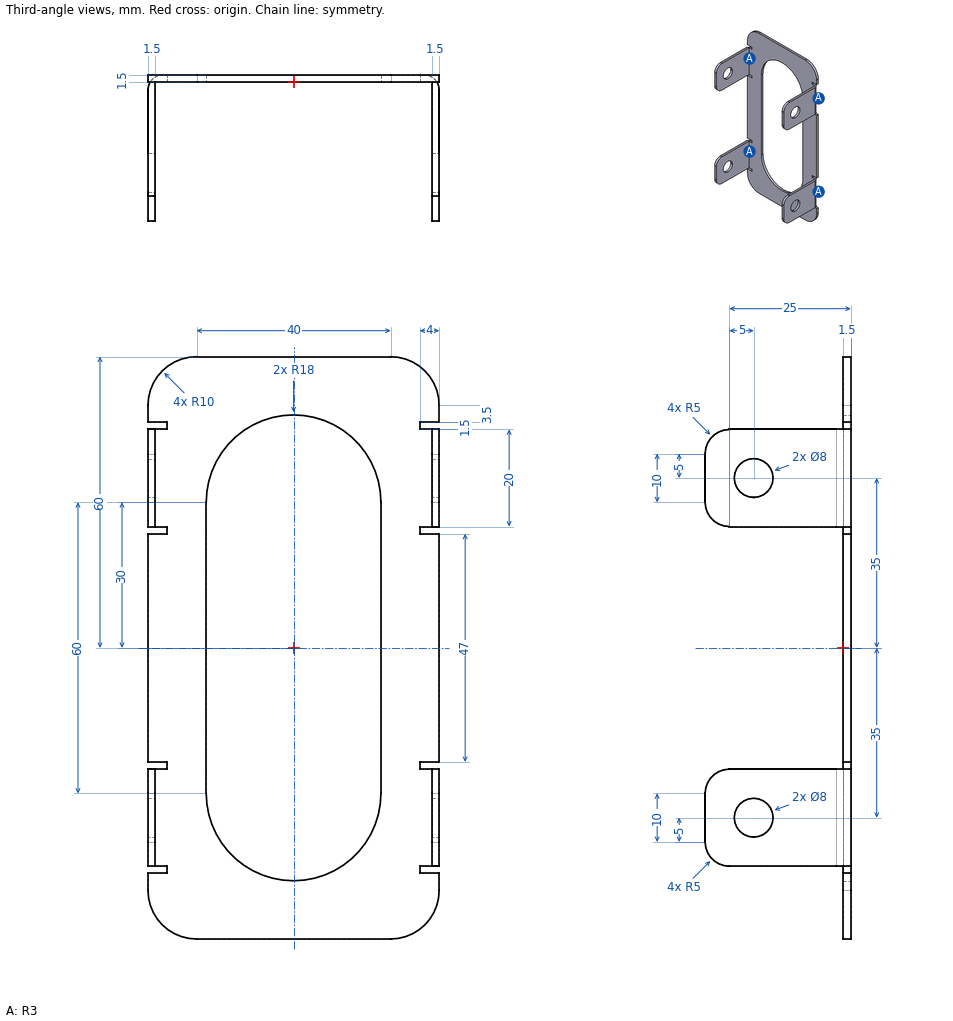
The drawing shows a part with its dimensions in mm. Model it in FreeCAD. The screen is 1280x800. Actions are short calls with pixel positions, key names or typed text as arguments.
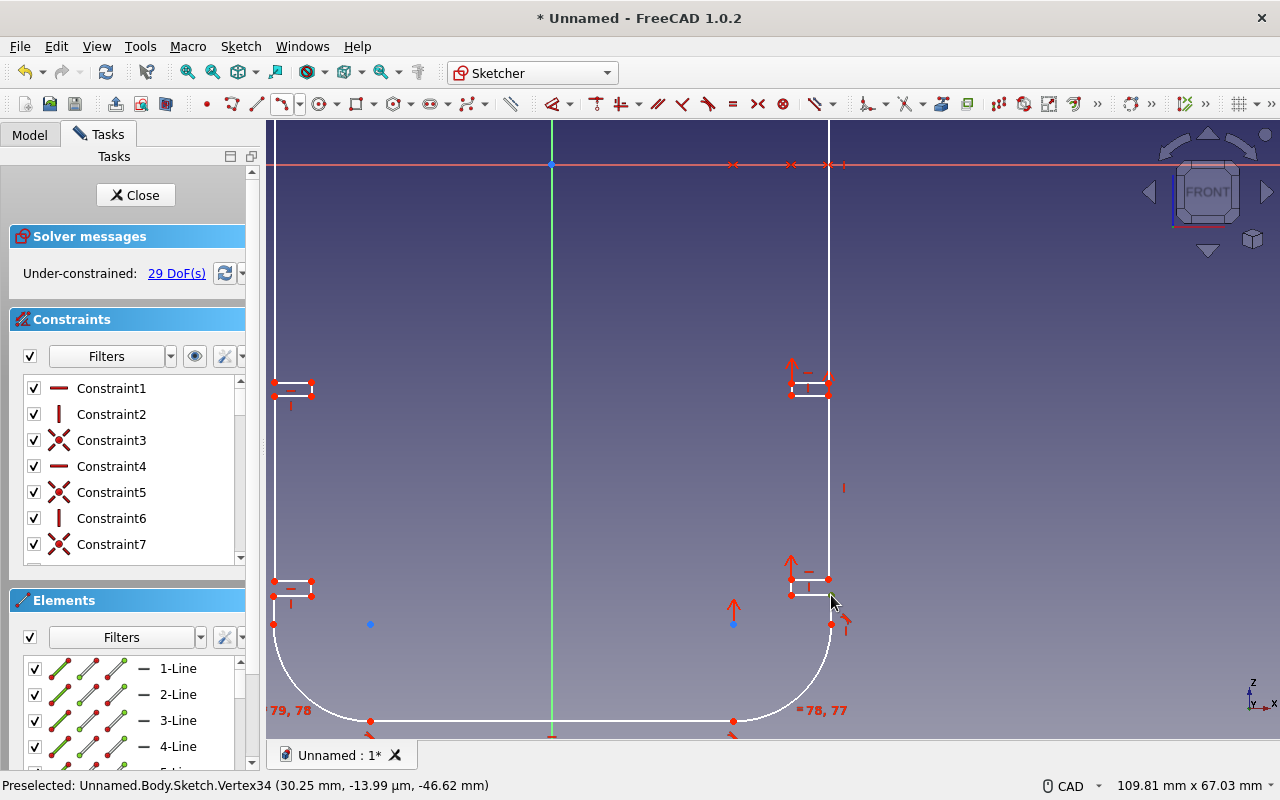
scroll(793, 584, down, 5)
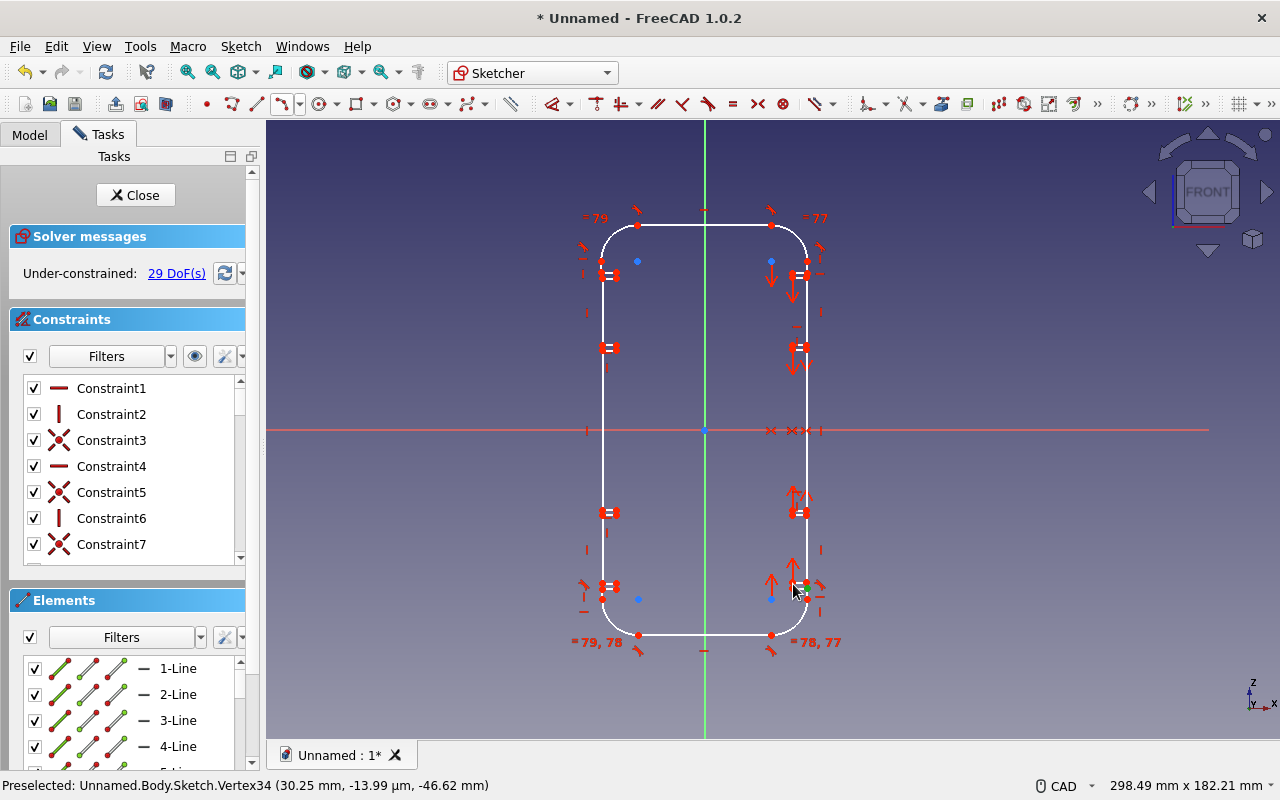
scroll(602, 589, up, 5)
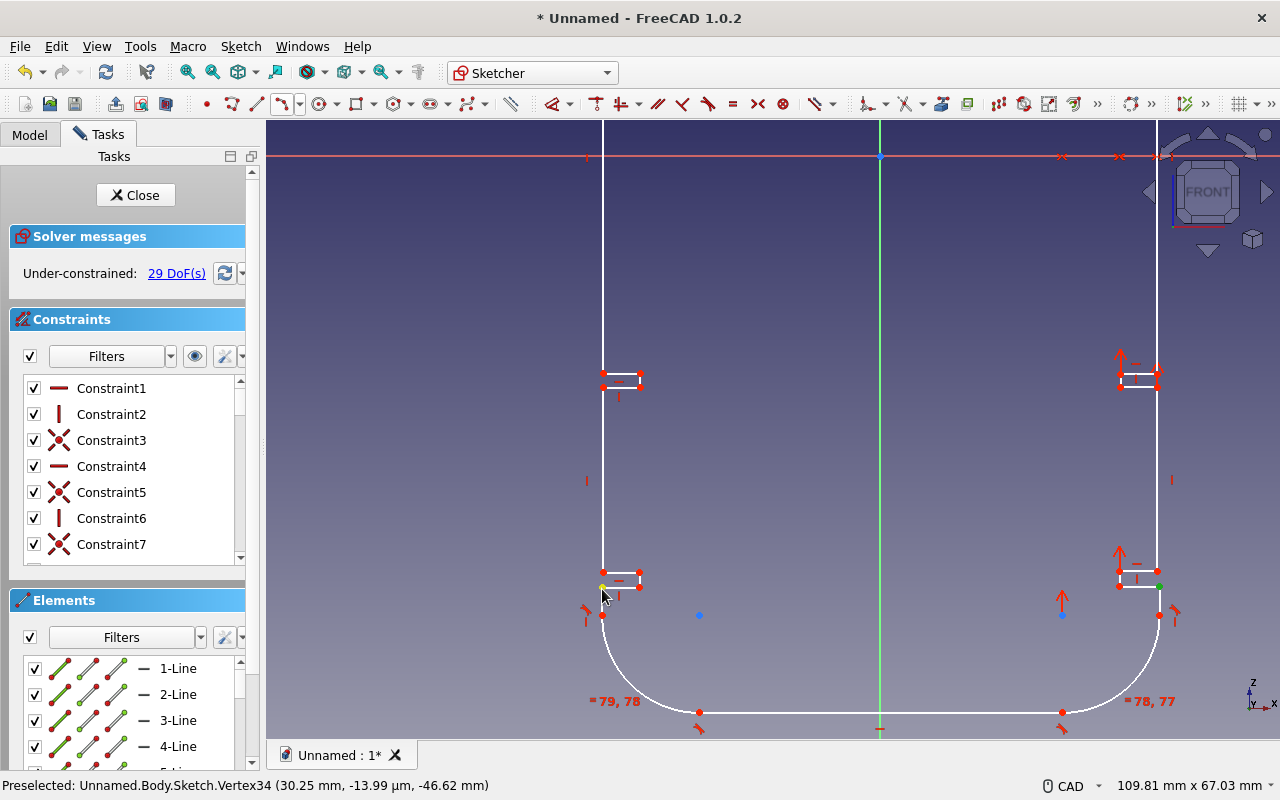
click(602, 588)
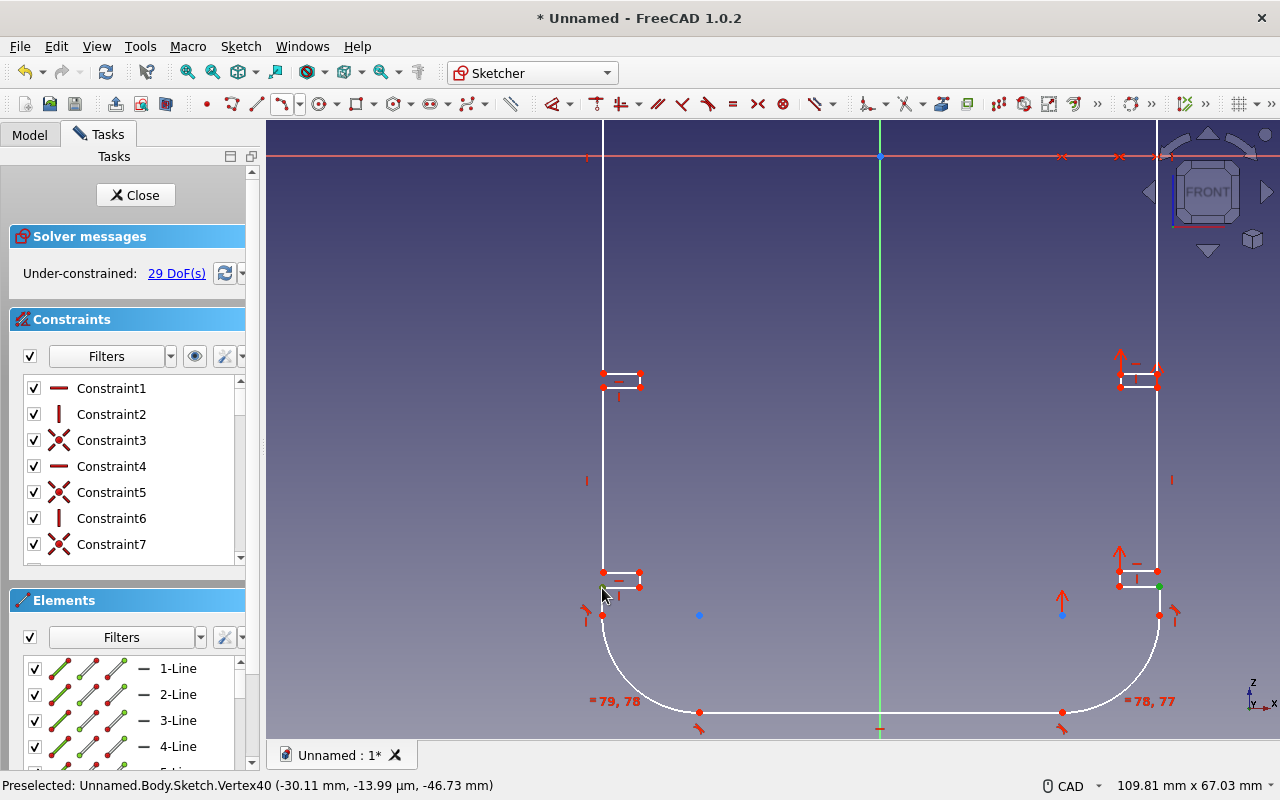
click(880, 671)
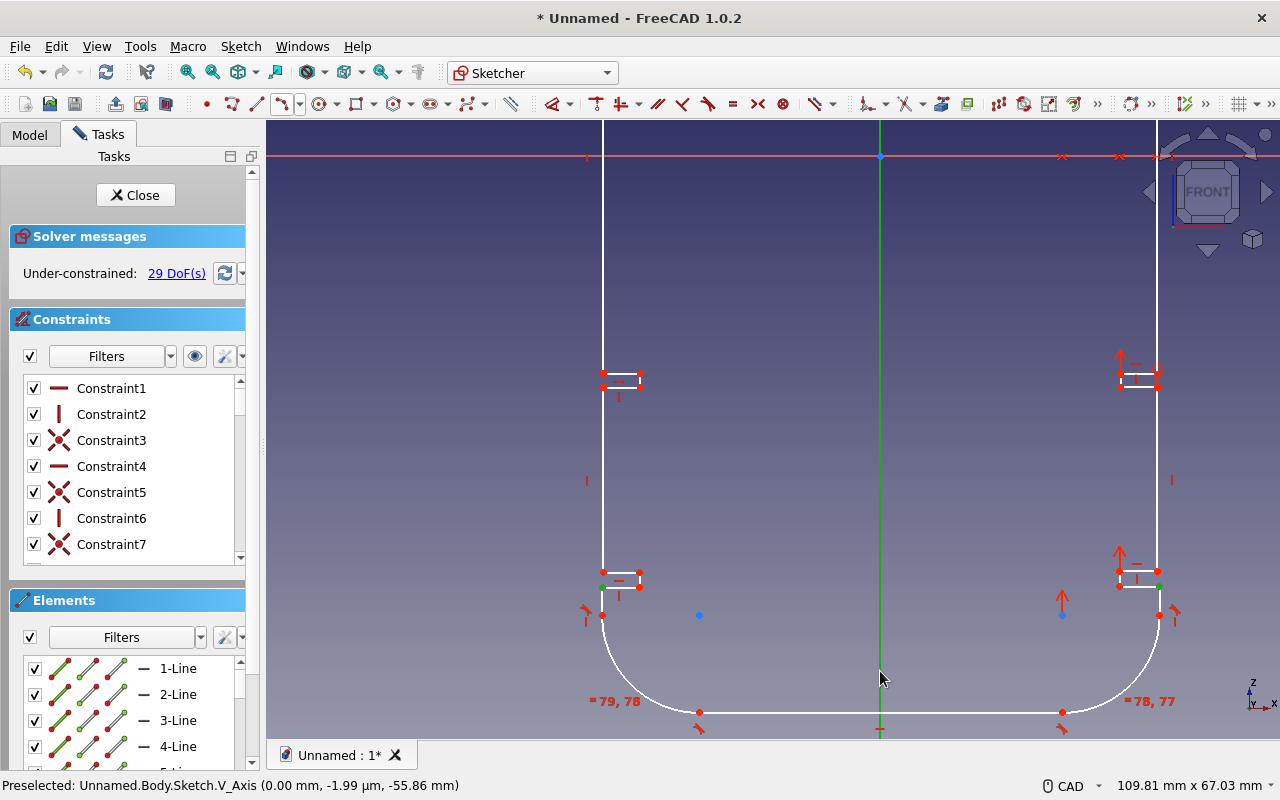
key(s)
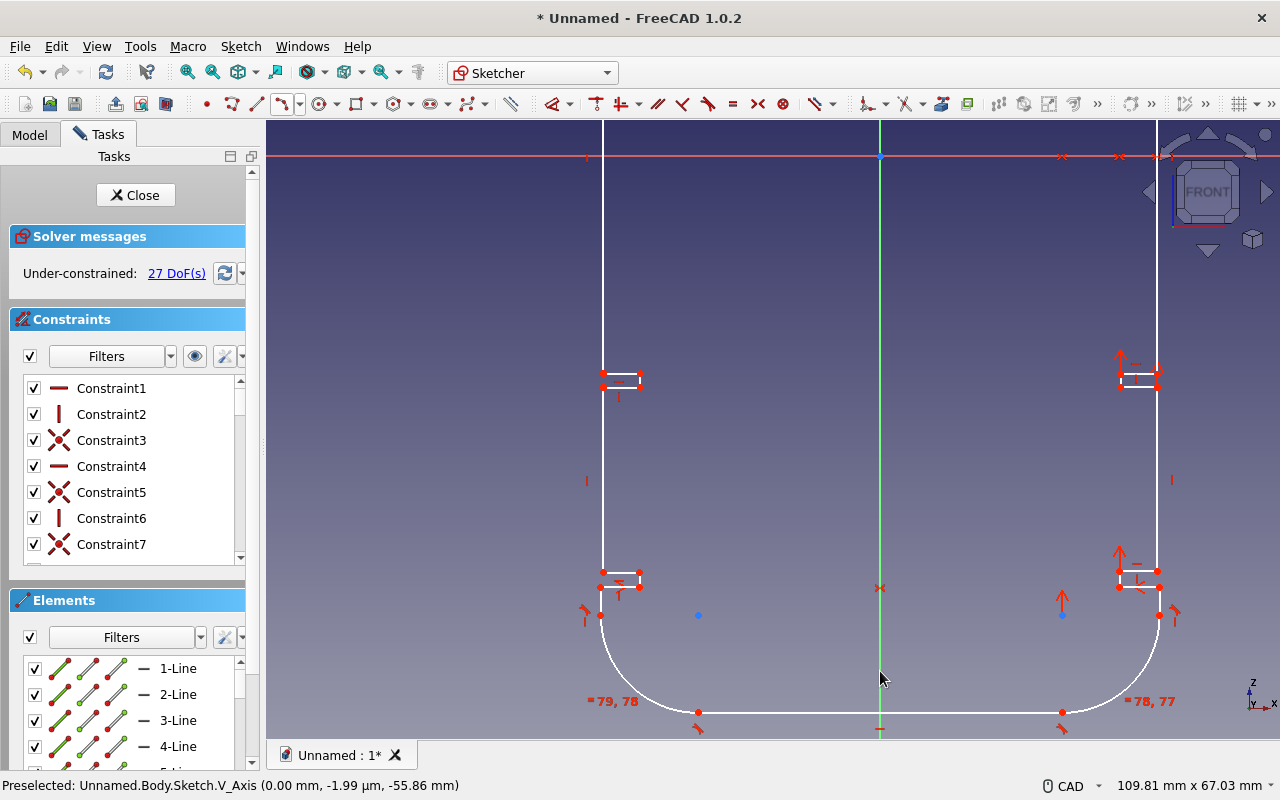
scroll(602, 589, down, 5)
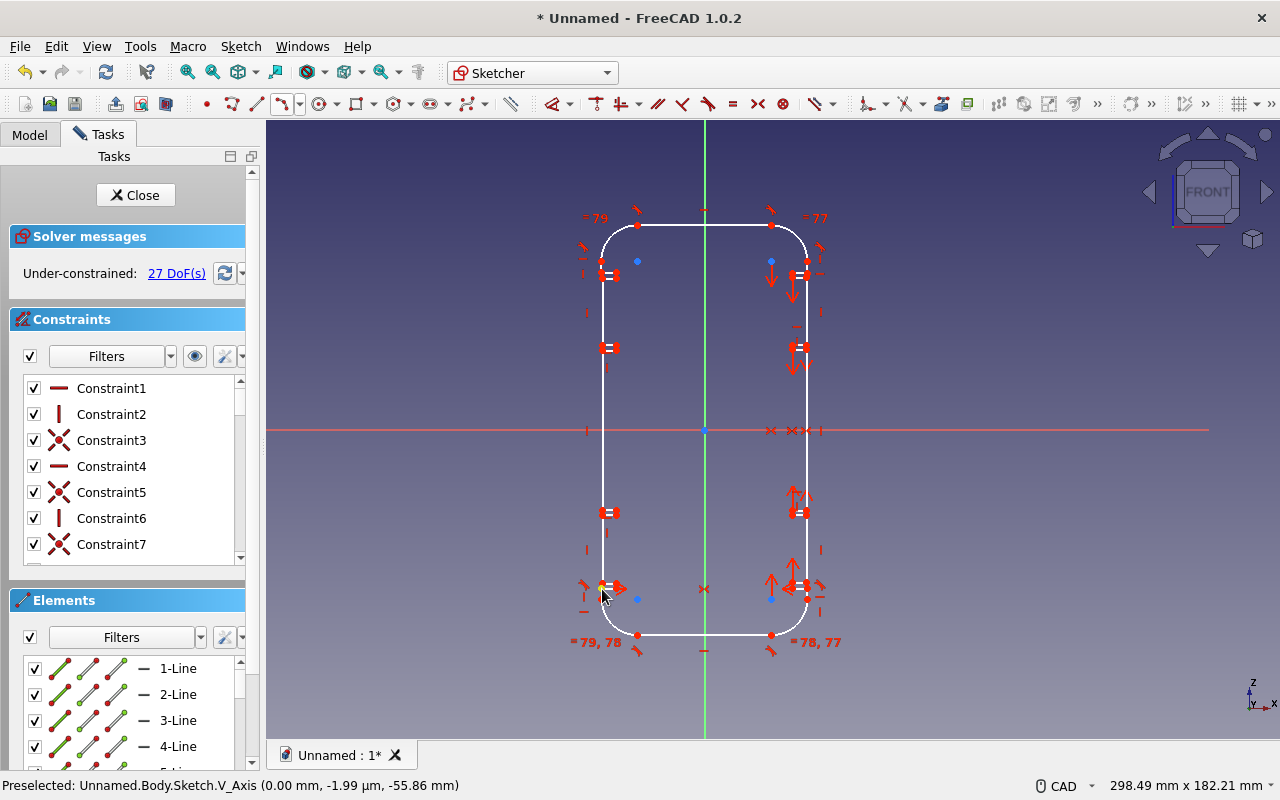
scroll(793, 583, up, 4)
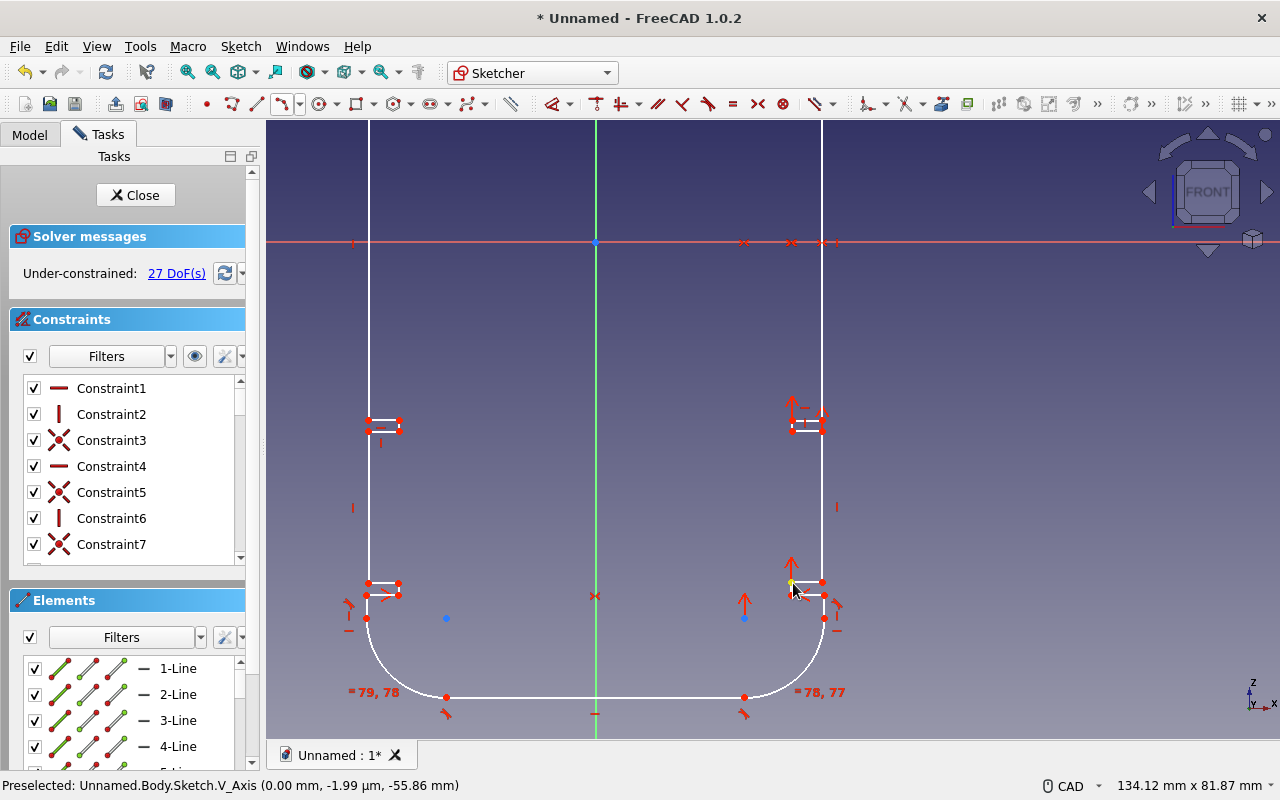
click(791, 582)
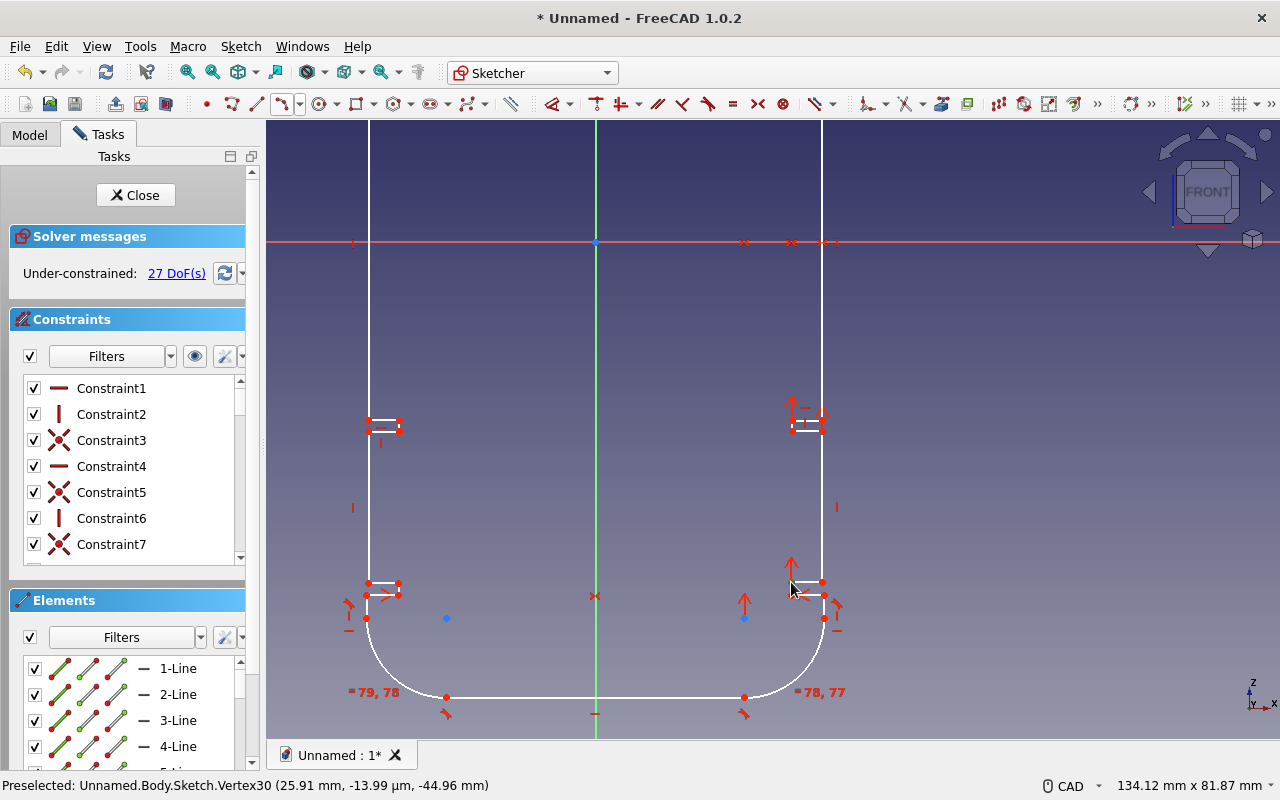
click(399, 583)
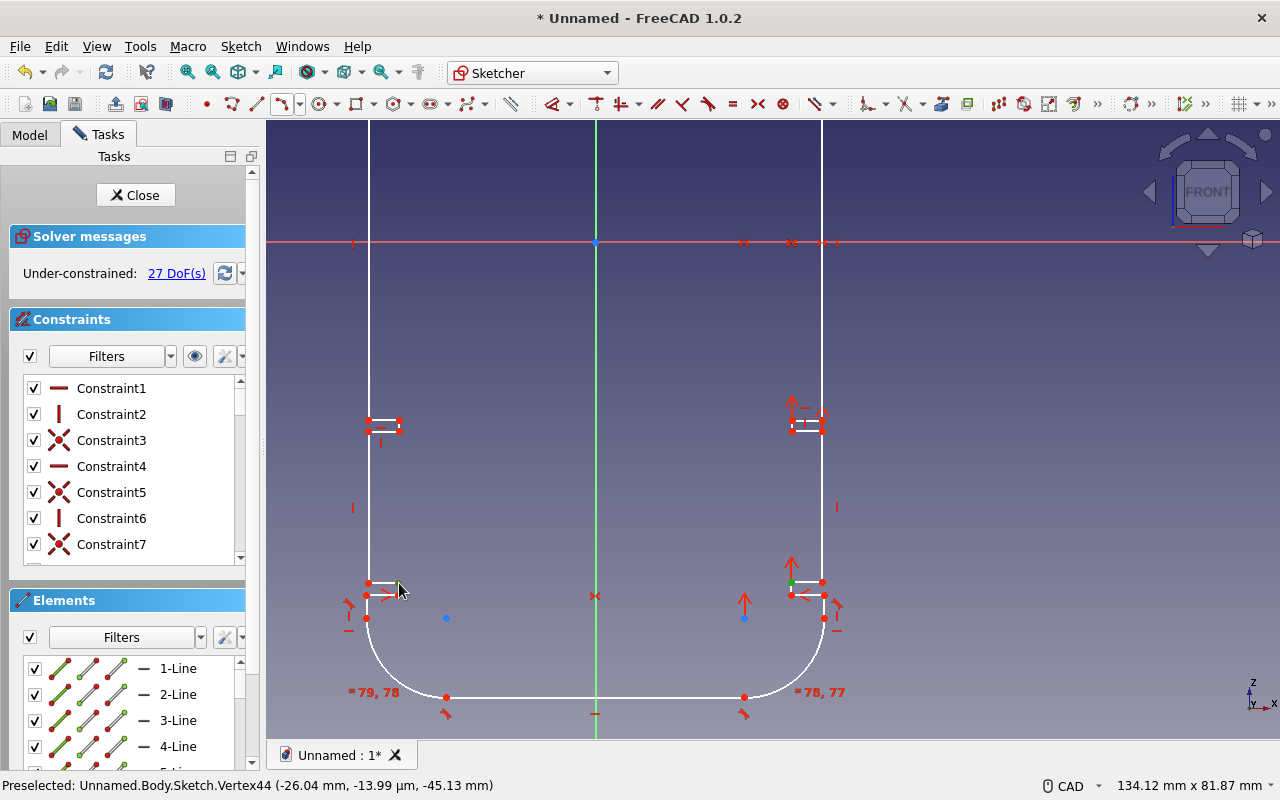
click(596, 631)